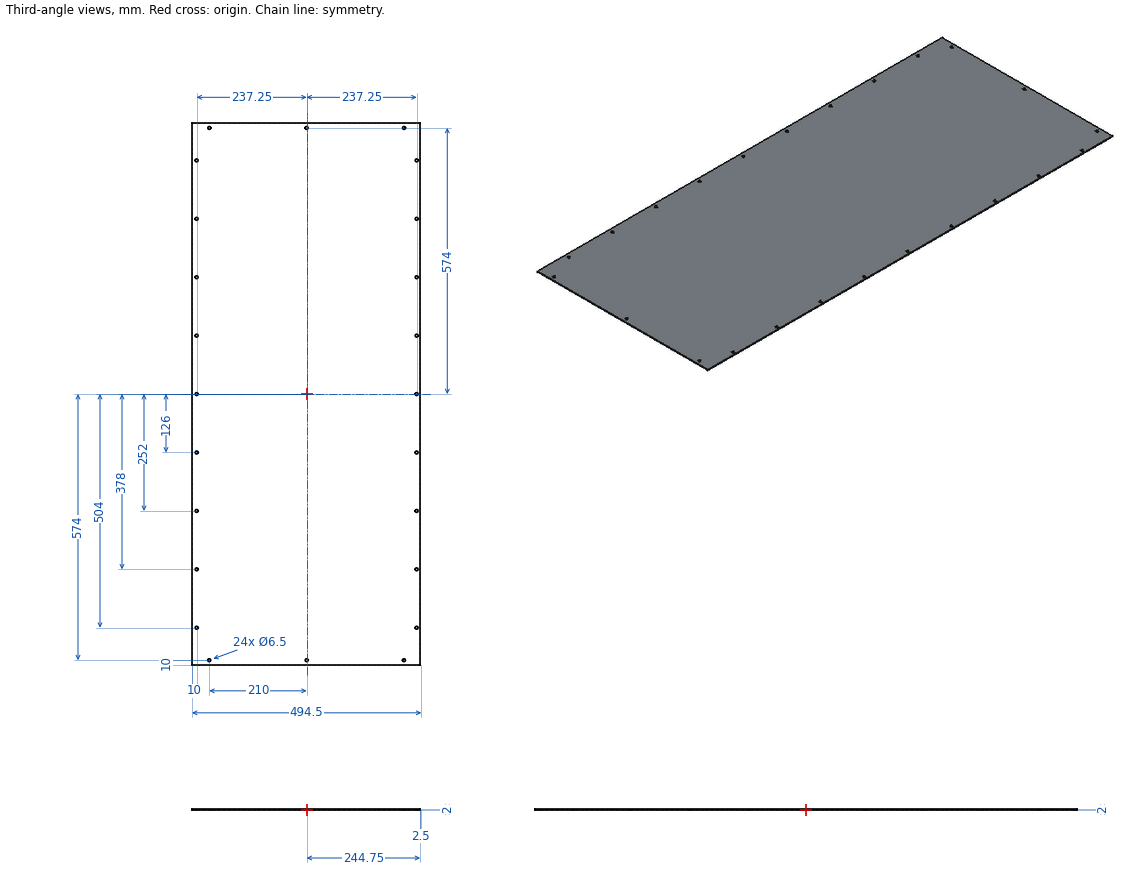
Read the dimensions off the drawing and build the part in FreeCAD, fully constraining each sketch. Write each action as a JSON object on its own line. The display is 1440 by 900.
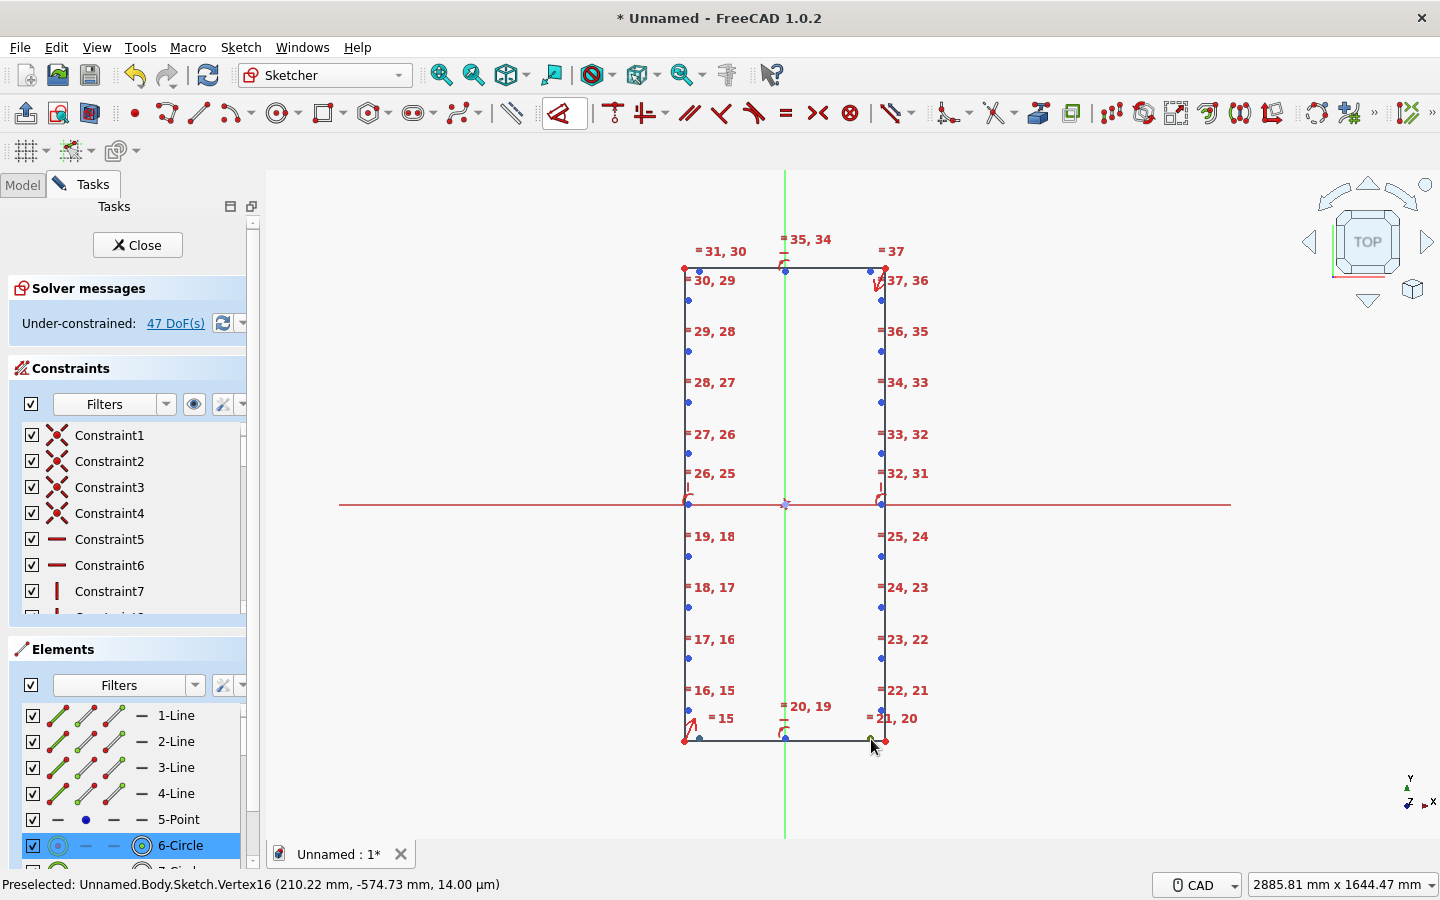
{"action": "left_click", "coordinate": [785, 680]}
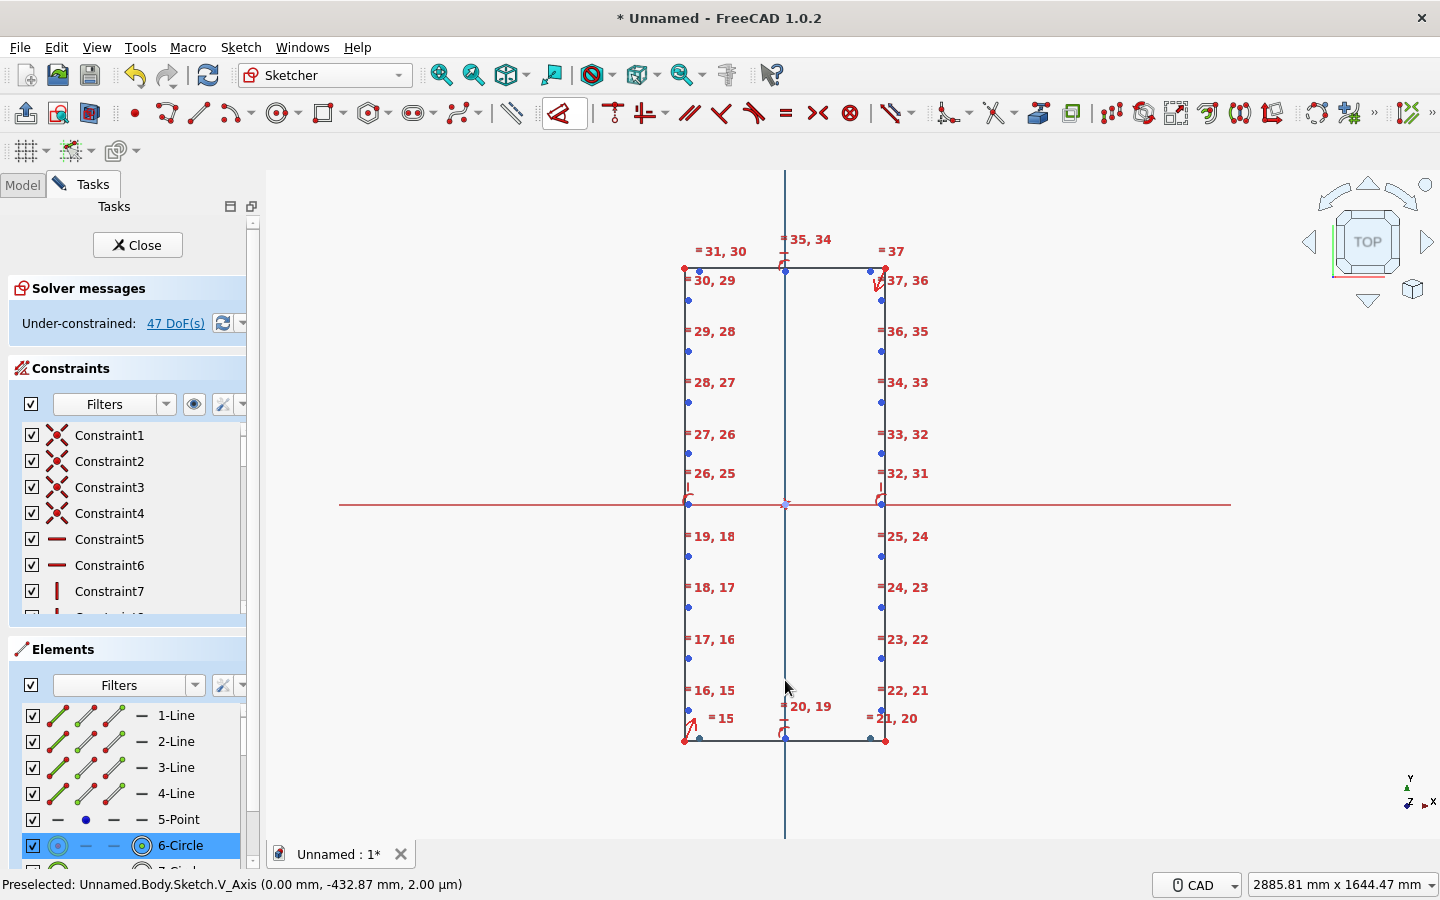
{"action": "left_click", "coordinate": [818, 114]}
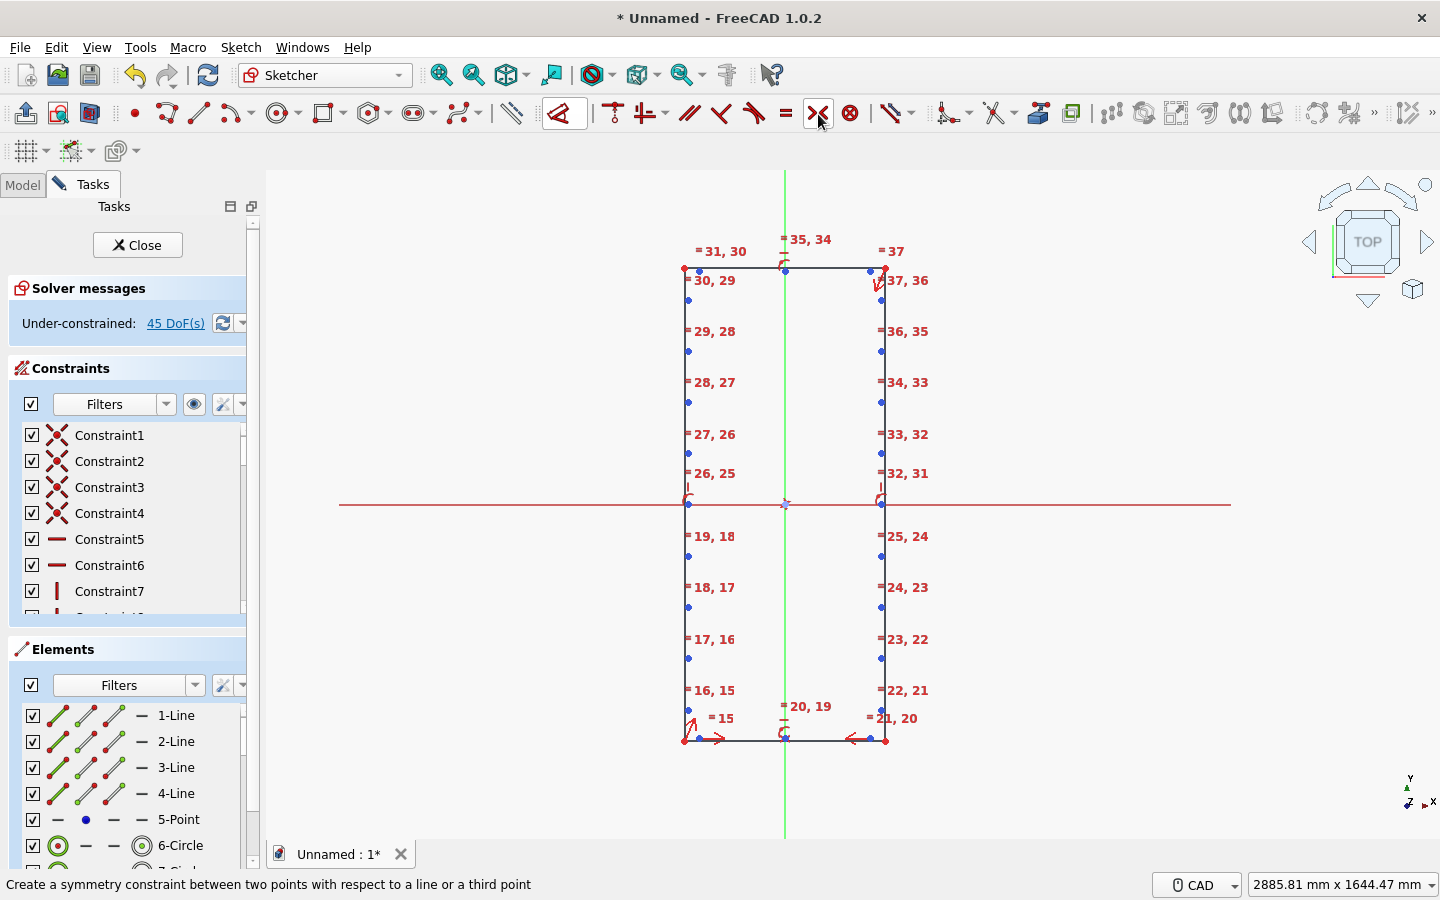
{"action": "left_click", "coordinate": [689, 710]}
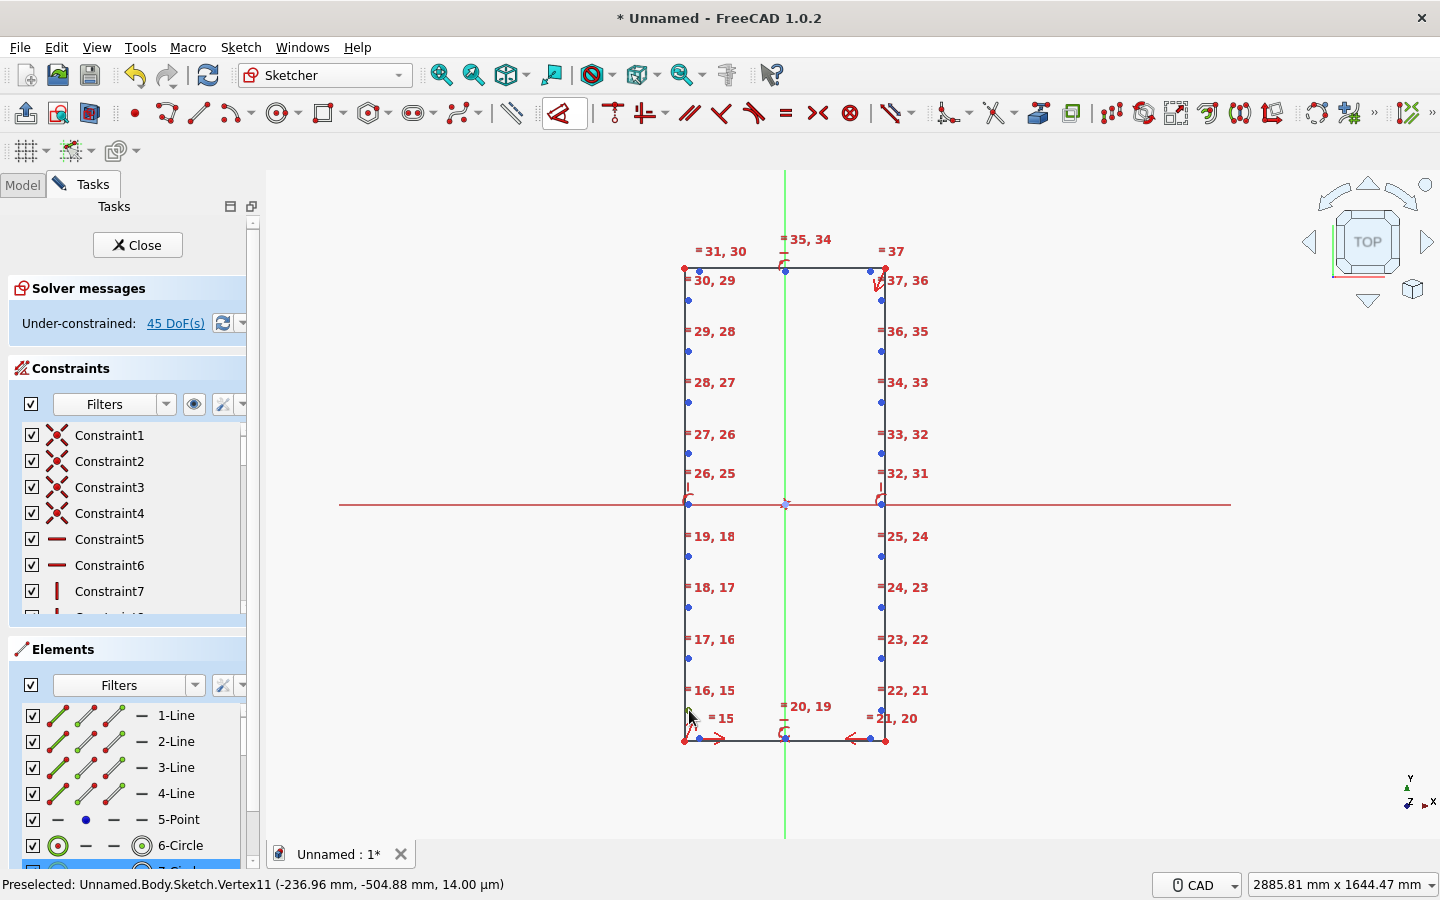
{"action": "left_click", "coordinate": [882, 710]}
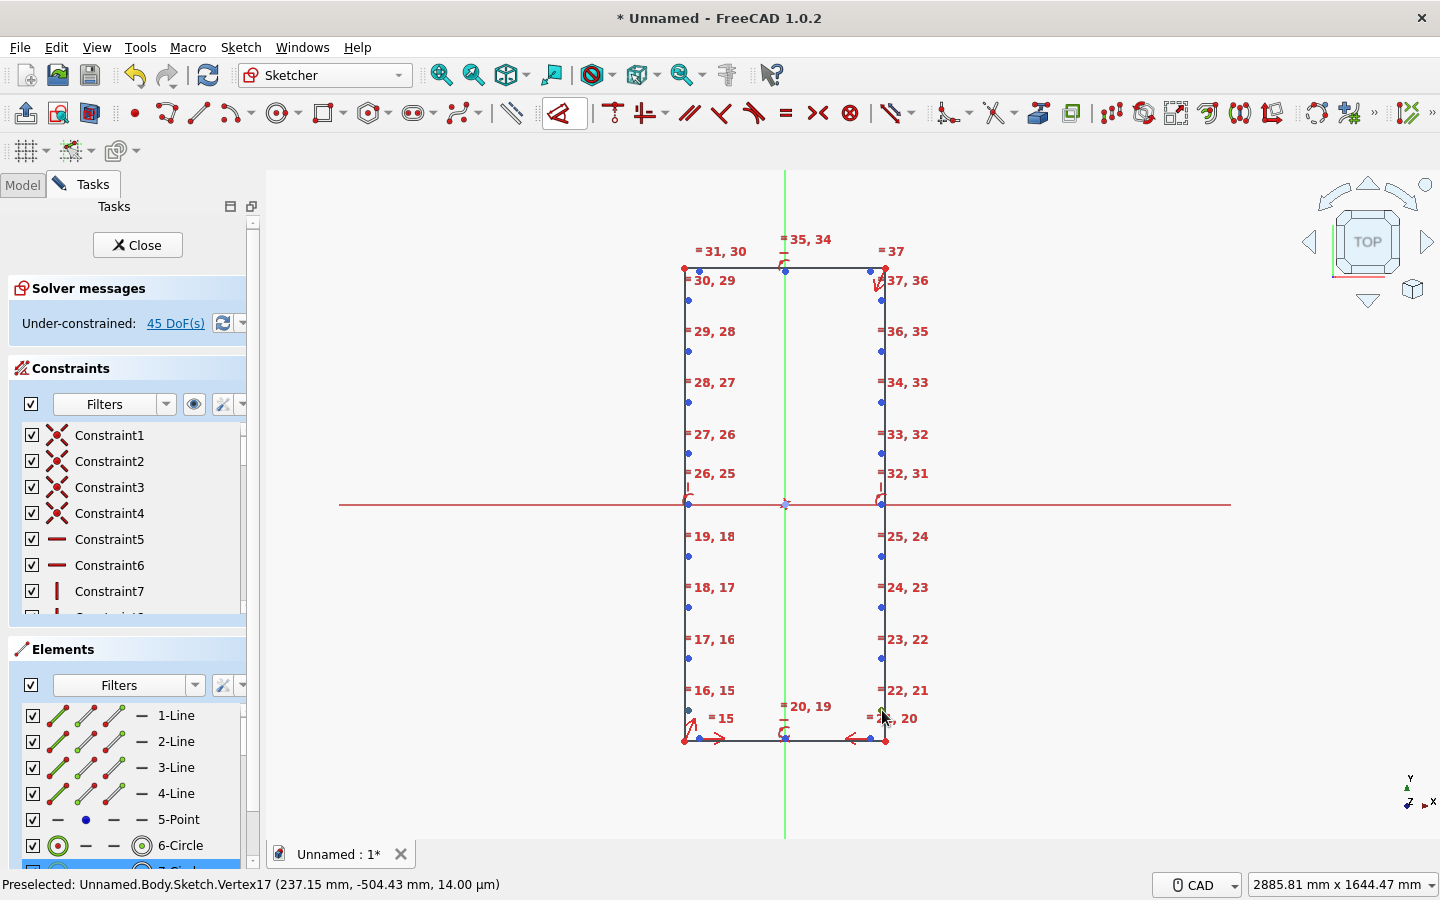
{"action": "left_click", "coordinate": [785, 680]}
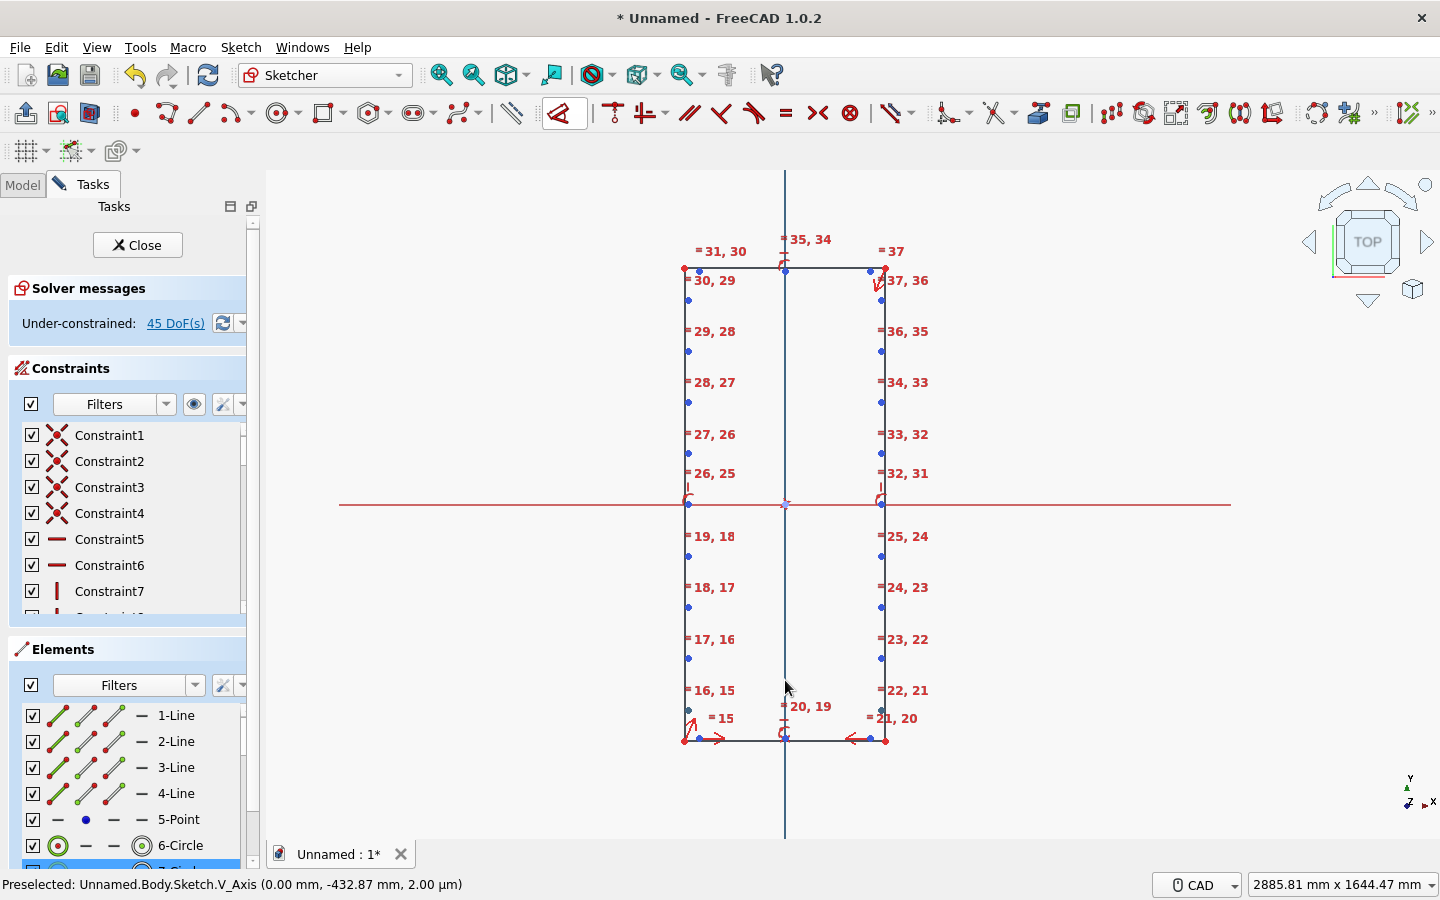
{"action": "key", "text": "s"}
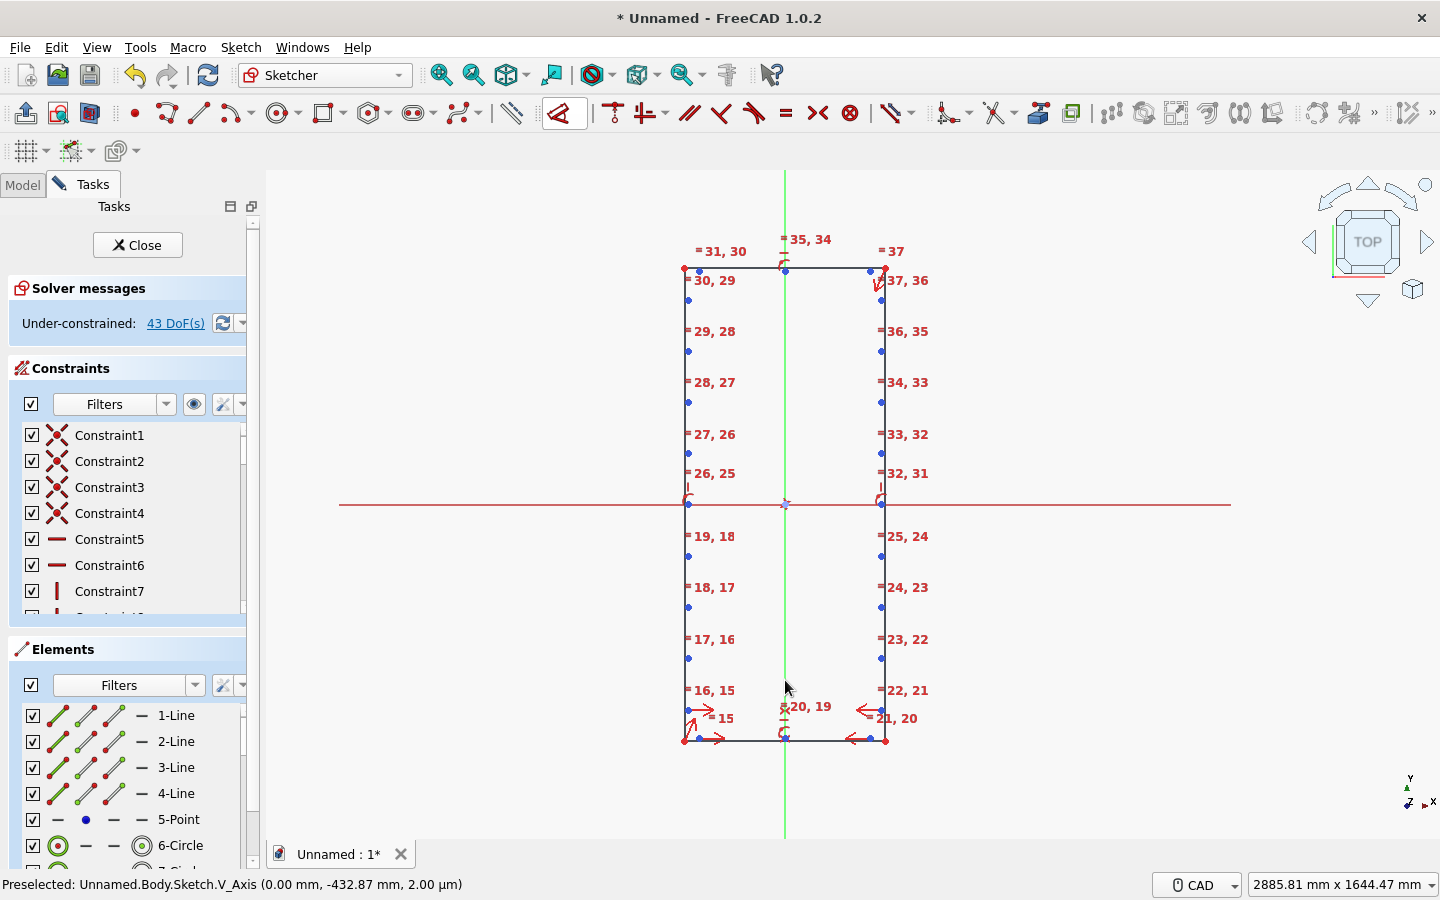
{"action": "left_click", "coordinate": [689, 659]}